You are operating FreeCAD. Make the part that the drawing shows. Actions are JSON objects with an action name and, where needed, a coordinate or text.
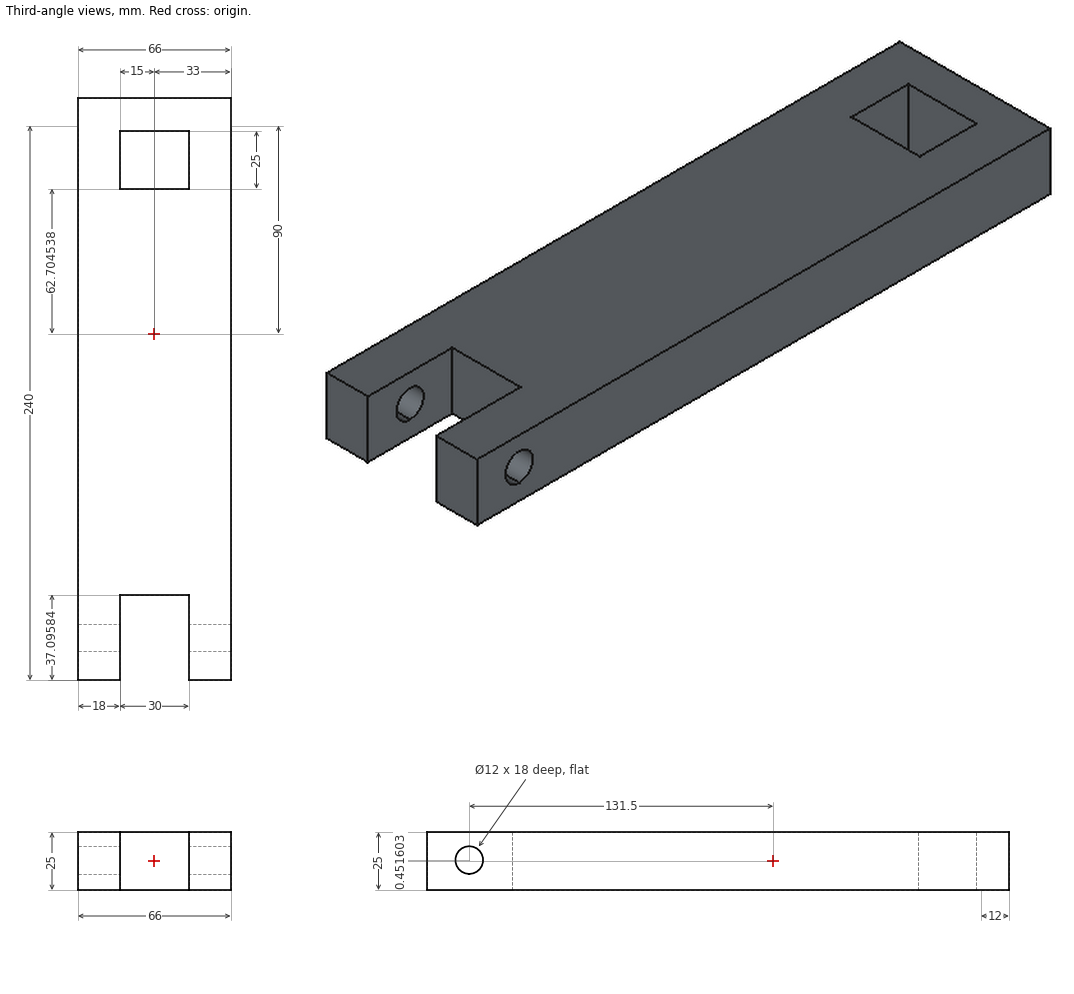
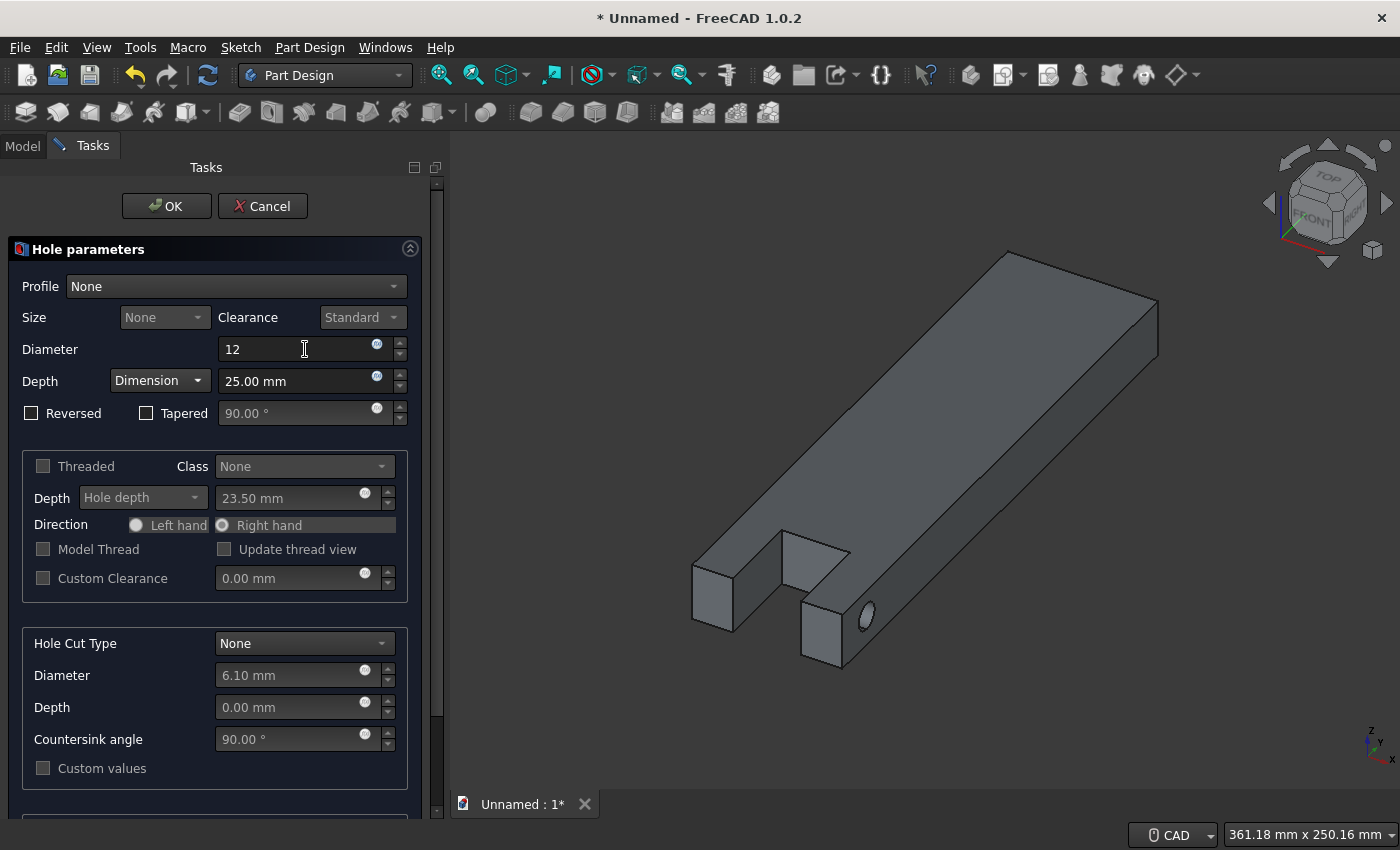
{"action": "triple_click", "coordinate": [305, 381]}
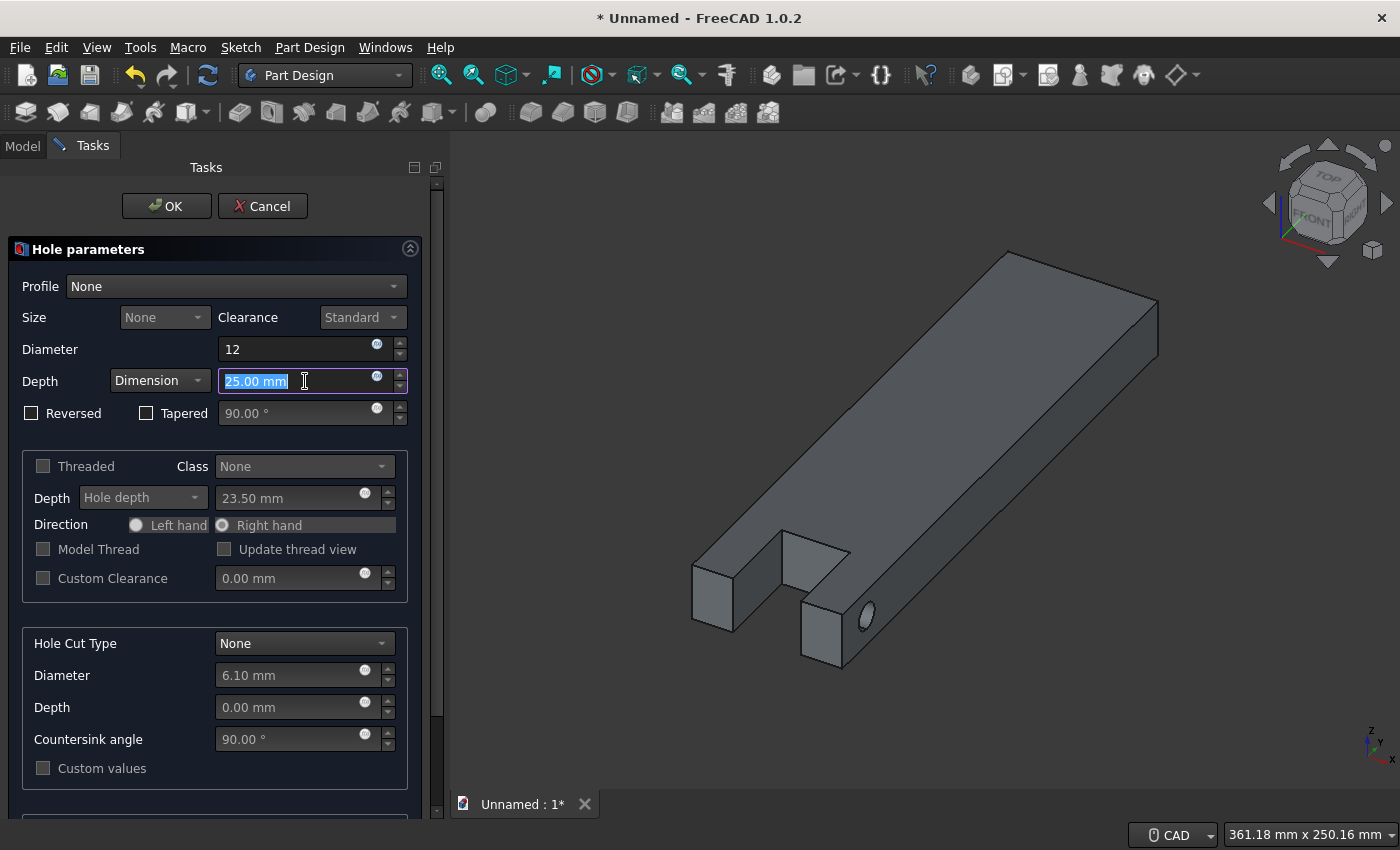
{"action": "type", "text": "18"}
{"action": "key", "text": "Tab"}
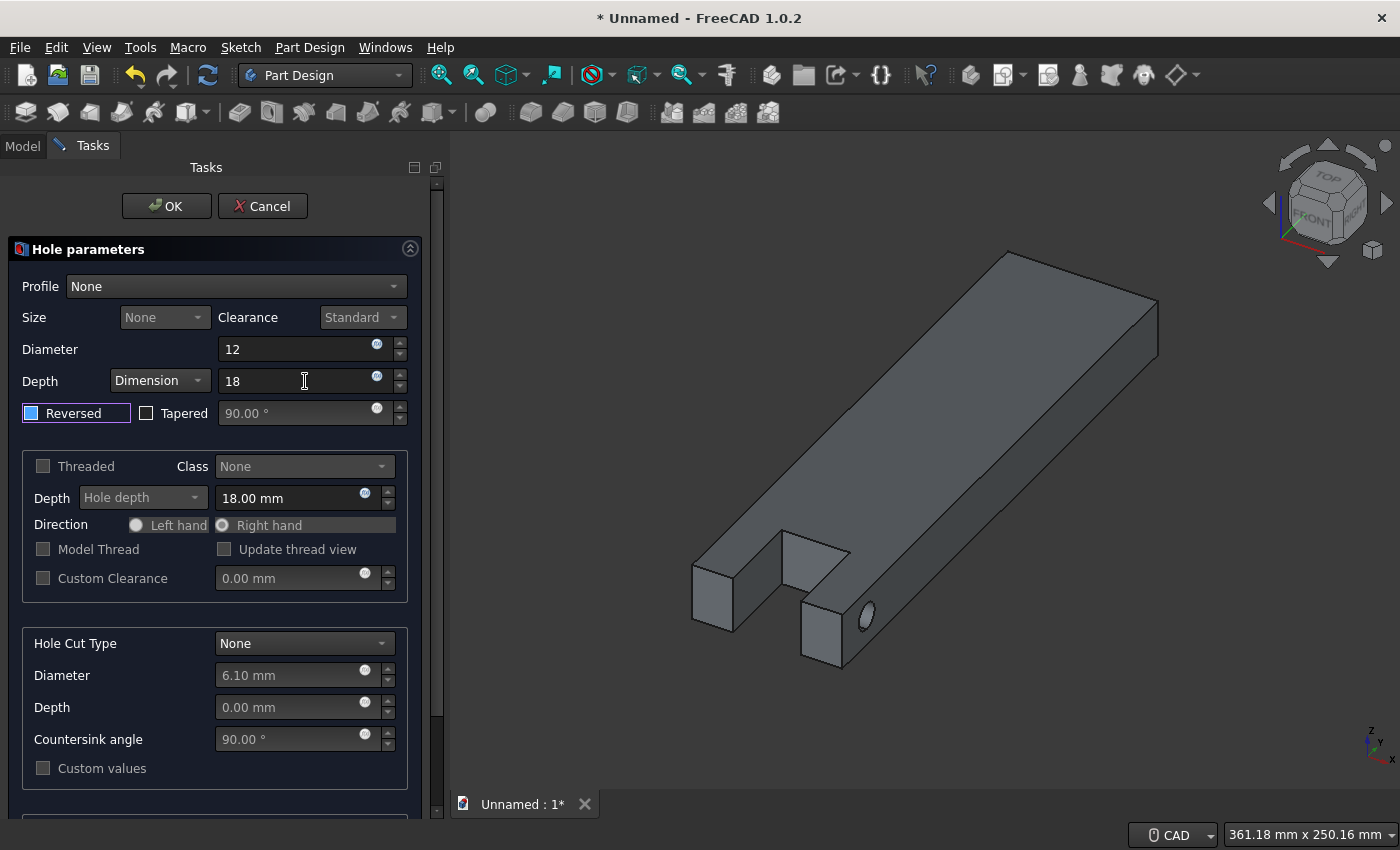
{"action": "scroll", "coordinate": [437, 498], "scroll_direction": "down", "scroll_amount": 2}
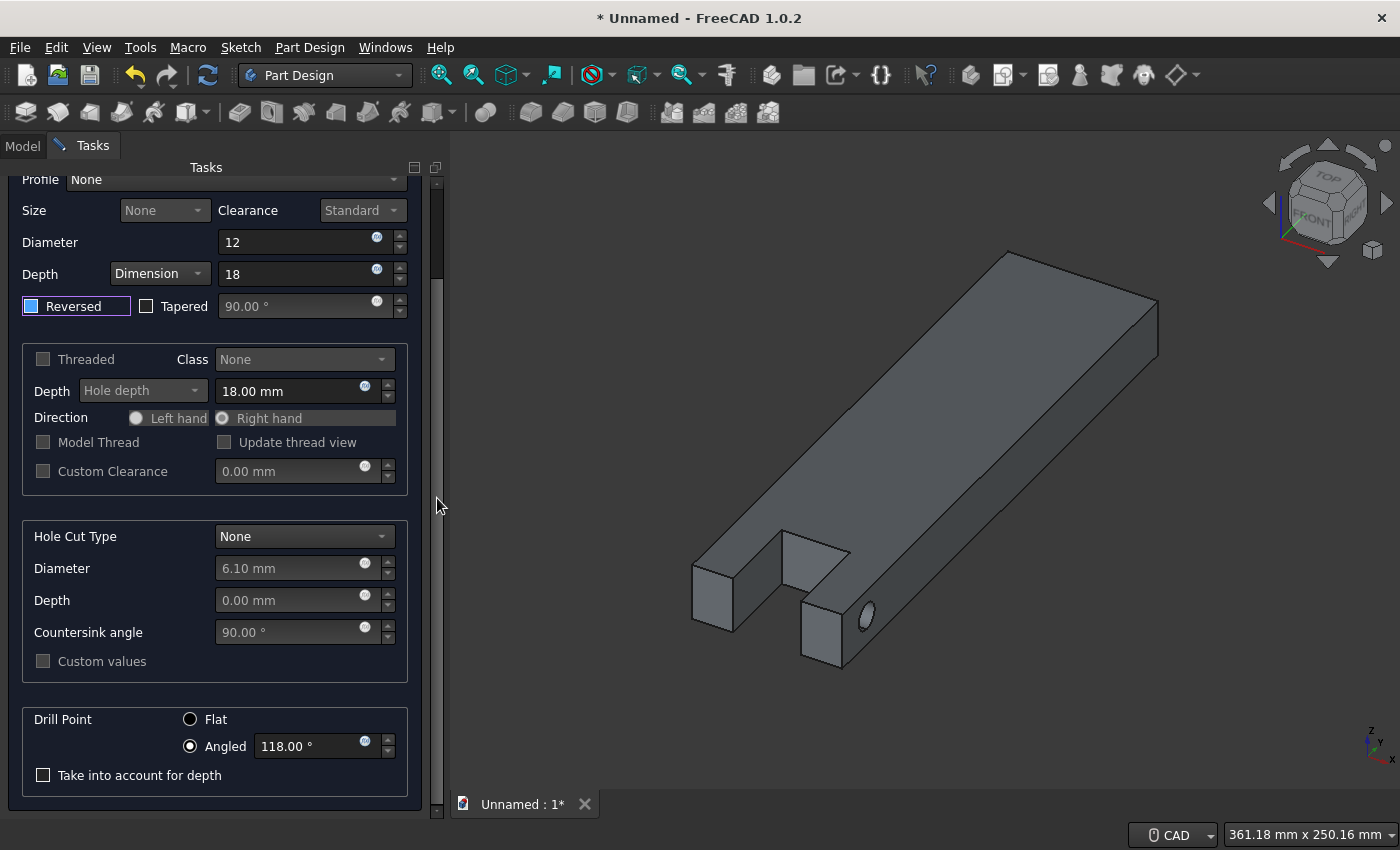
{"action": "left_click", "coordinate": [191, 719]}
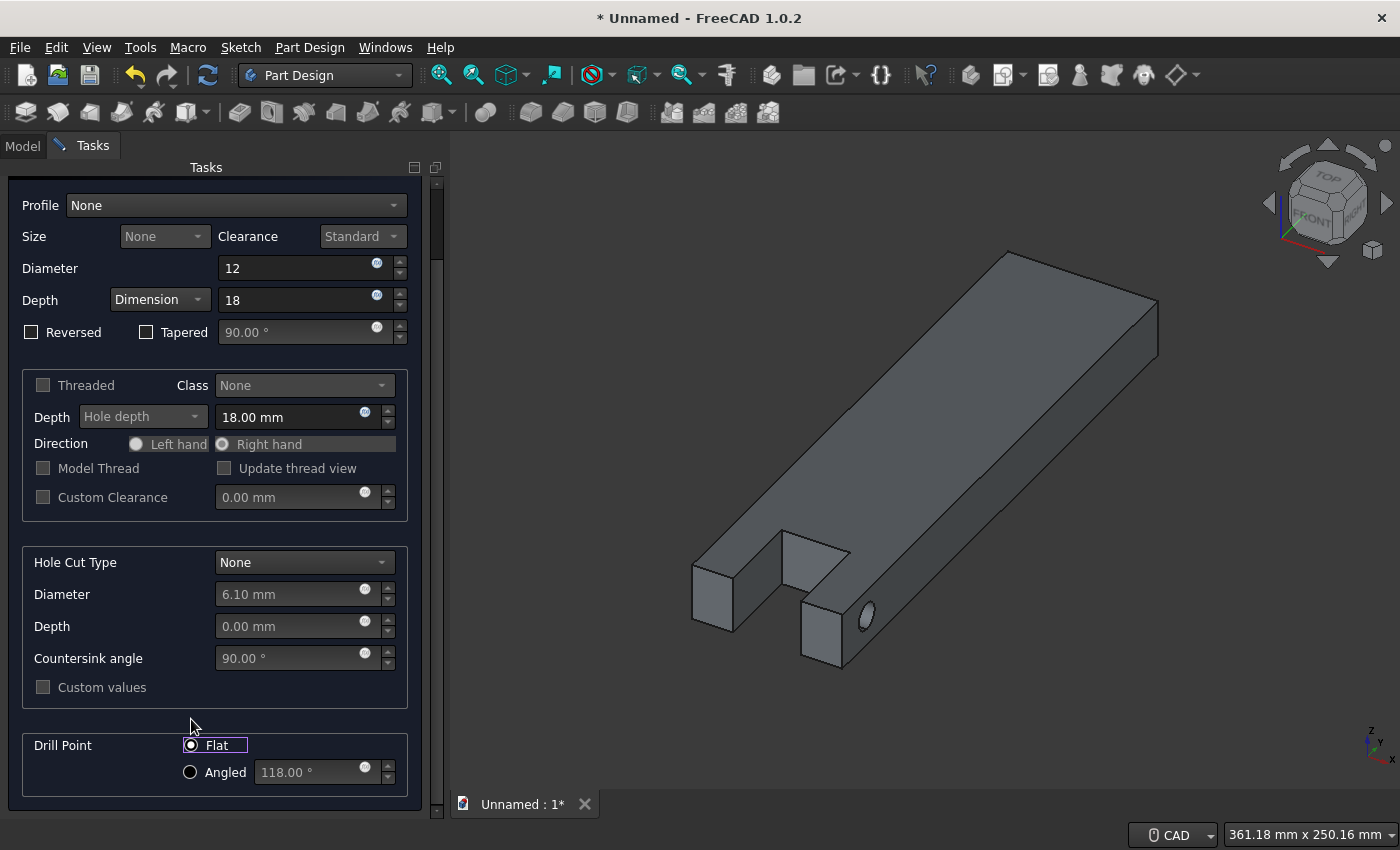
{"action": "scroll", "coordinate": [437, 498], "scroll_direction": "up", "scroll_amount": 3}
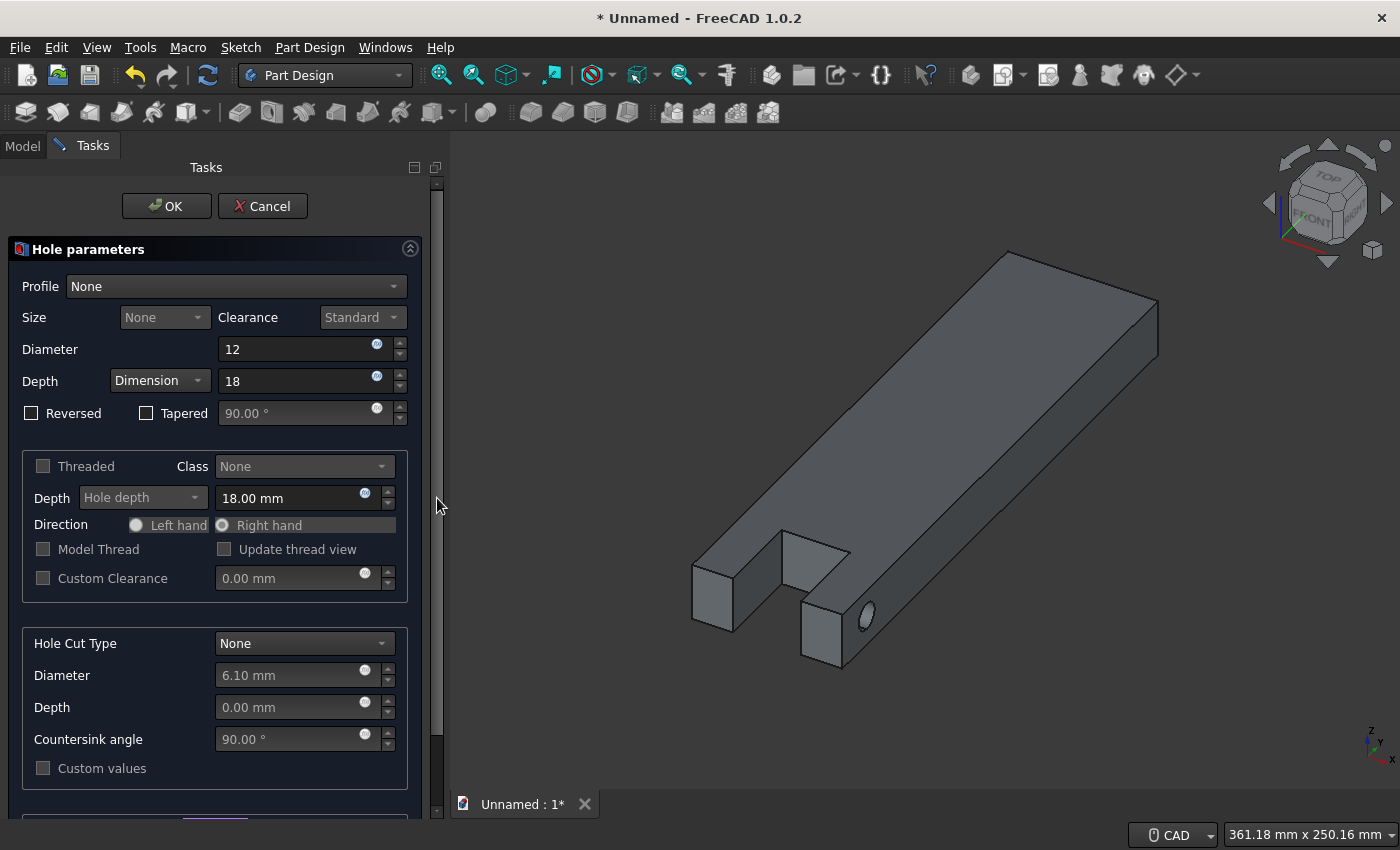
{"action": "left_click", "coordinate": [167, 206]}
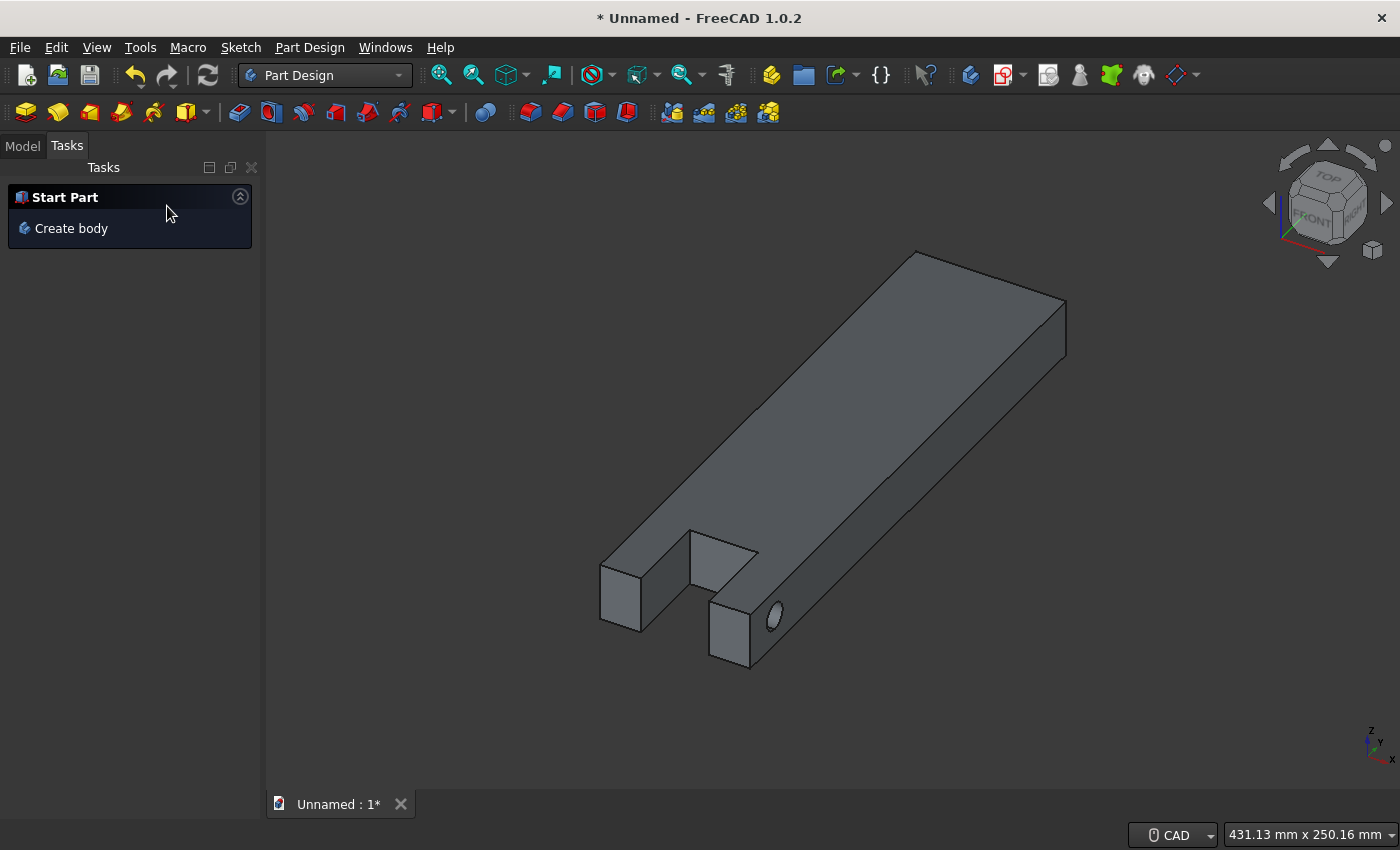
{"action": "left_click", "coordinate": [23, 145]}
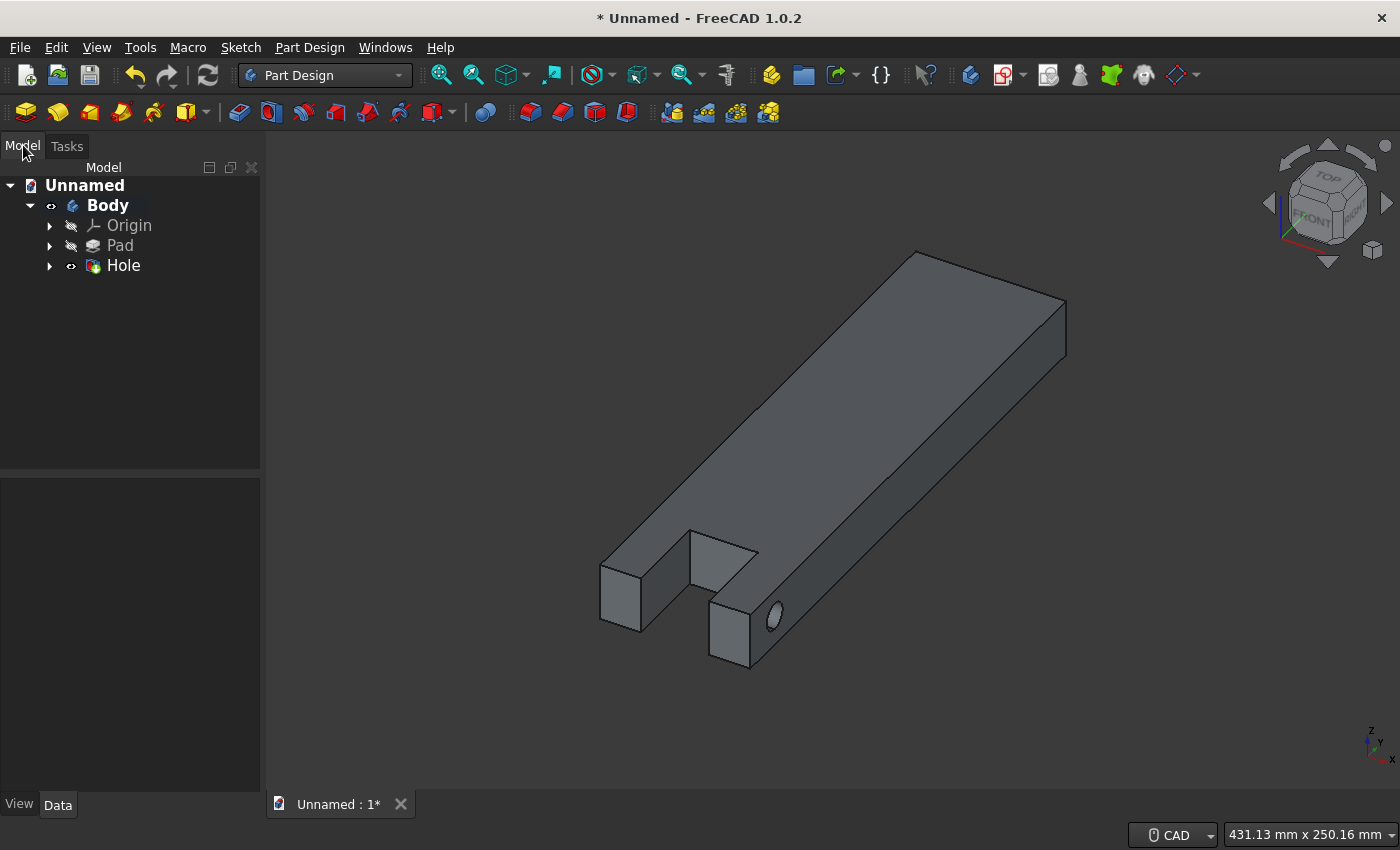
{"action": "left_click", "coordinate": [116, 266]}